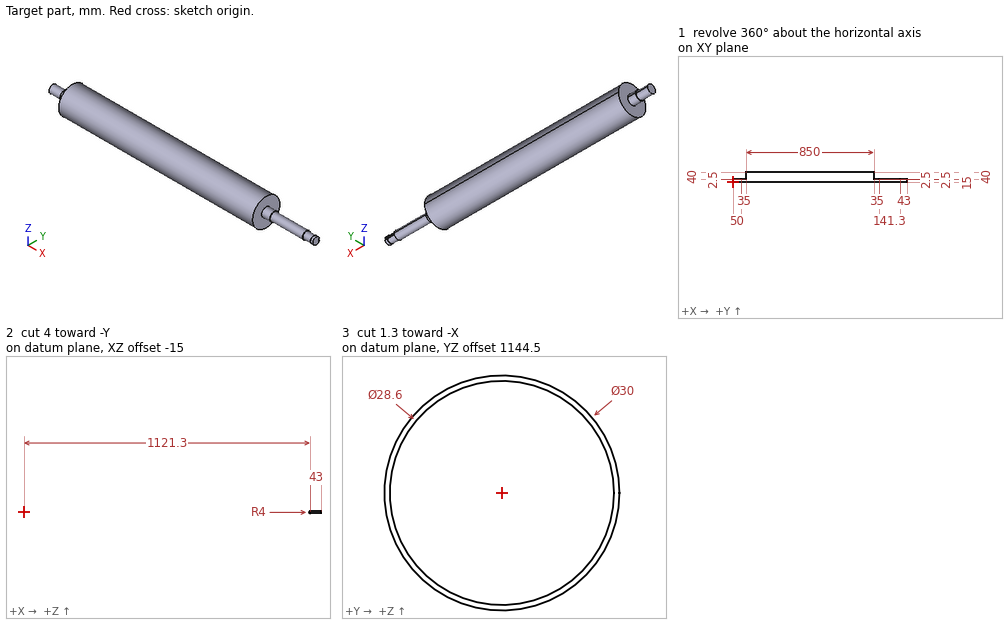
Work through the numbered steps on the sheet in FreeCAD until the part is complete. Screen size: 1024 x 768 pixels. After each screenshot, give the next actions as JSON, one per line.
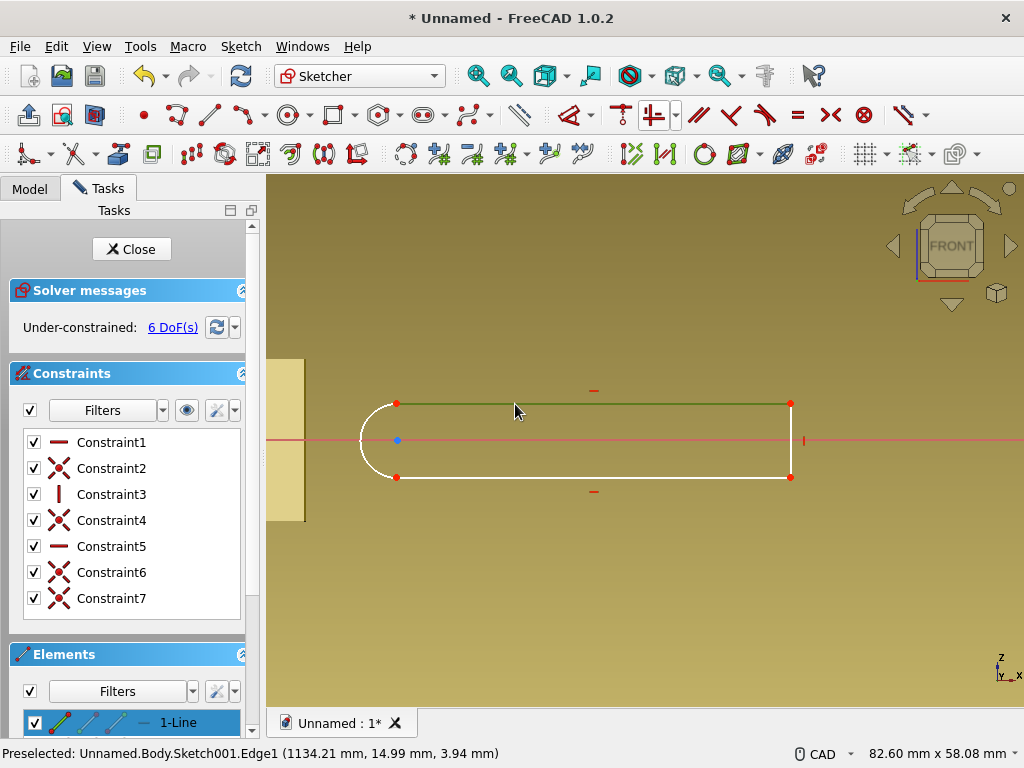
{"action": "left_click", "coordinate": [367, 419]}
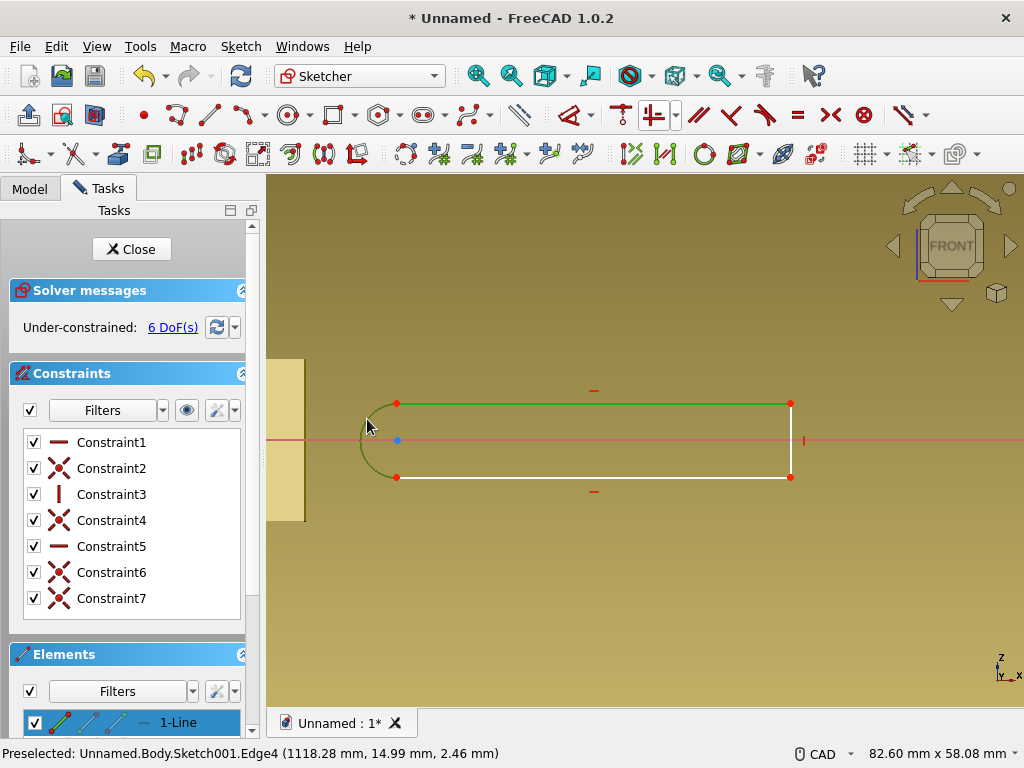
{"action": "left_click", "coordinate": [765, 116]}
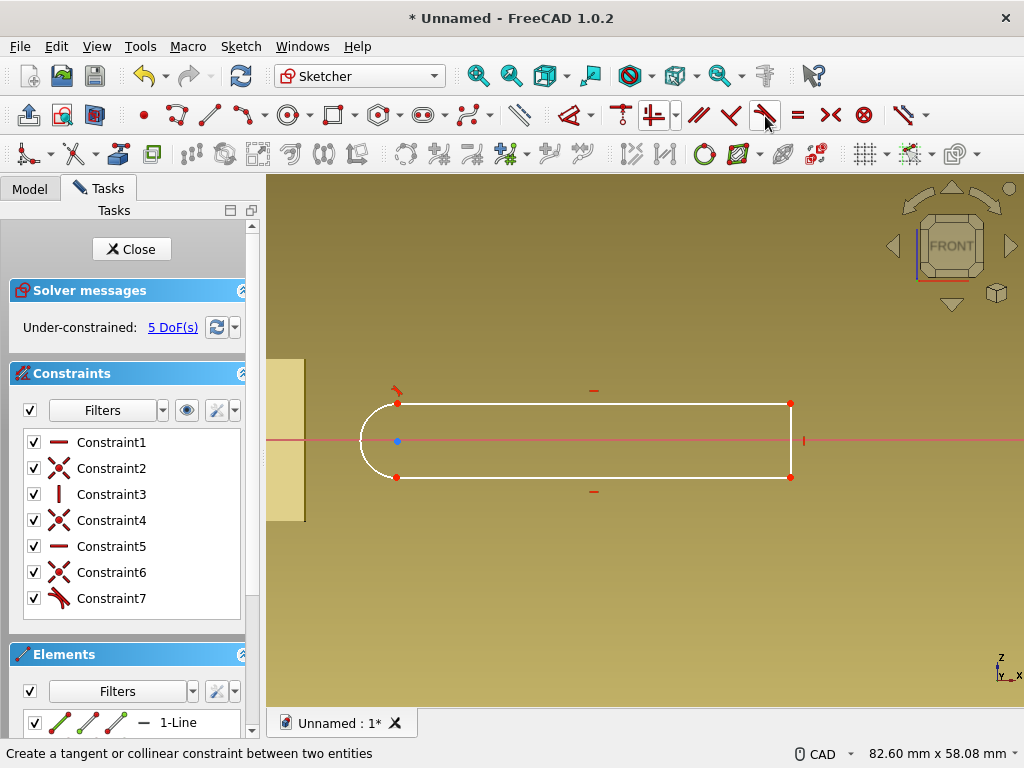
{"action": "left_click", "coordinate": [673, 478]}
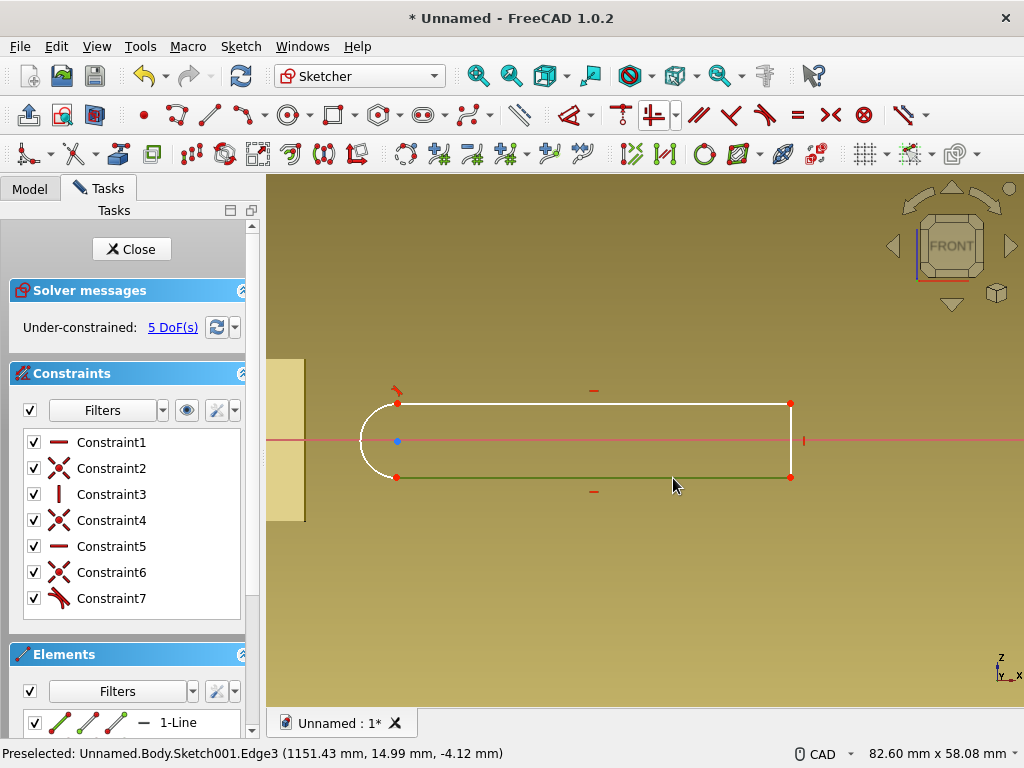
{"action": "left_click", "coordinate": [368, 419]}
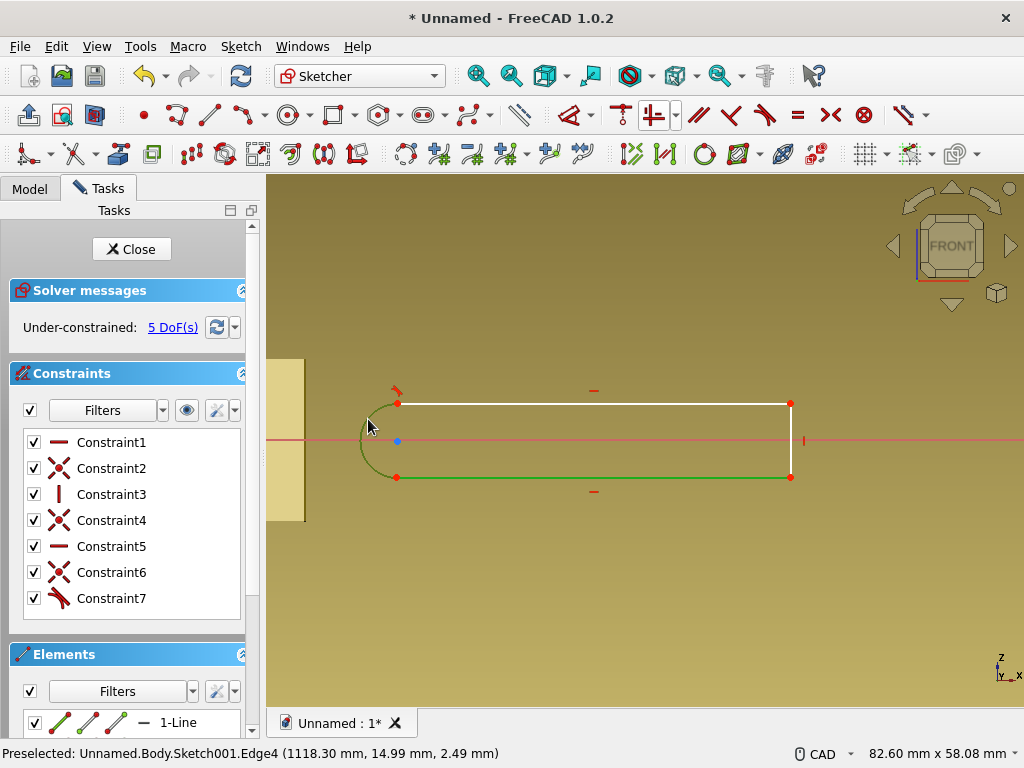
{"action": "key", "text": "t"}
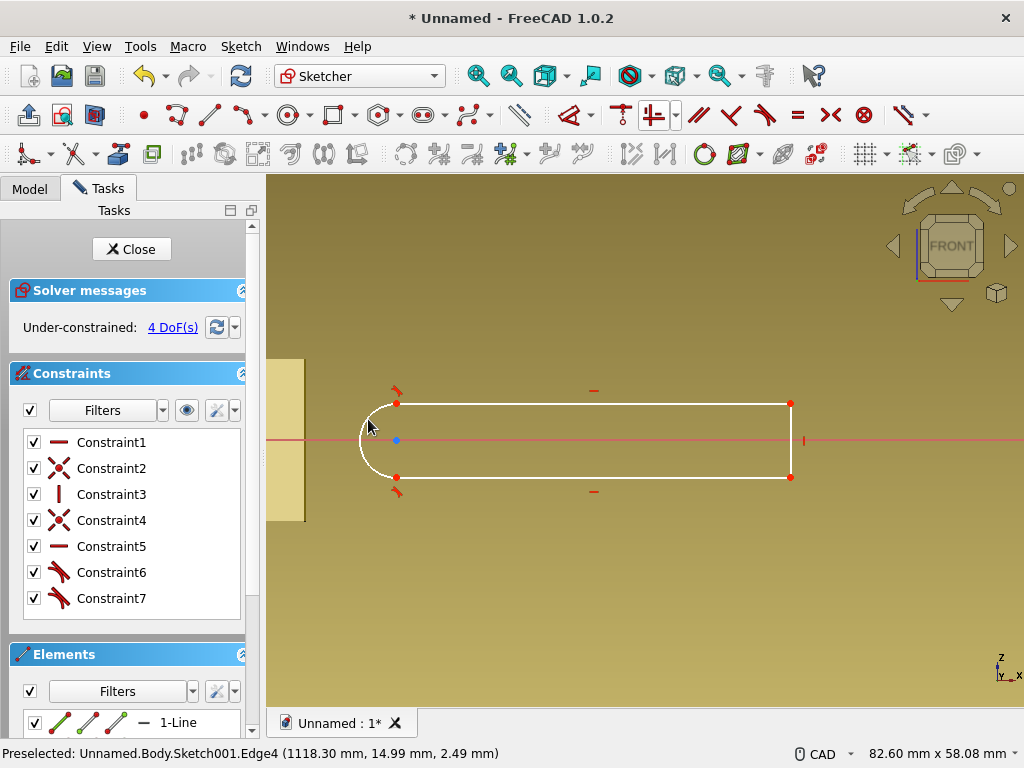
{"action": "left_click", "coordinate": [397, 441]}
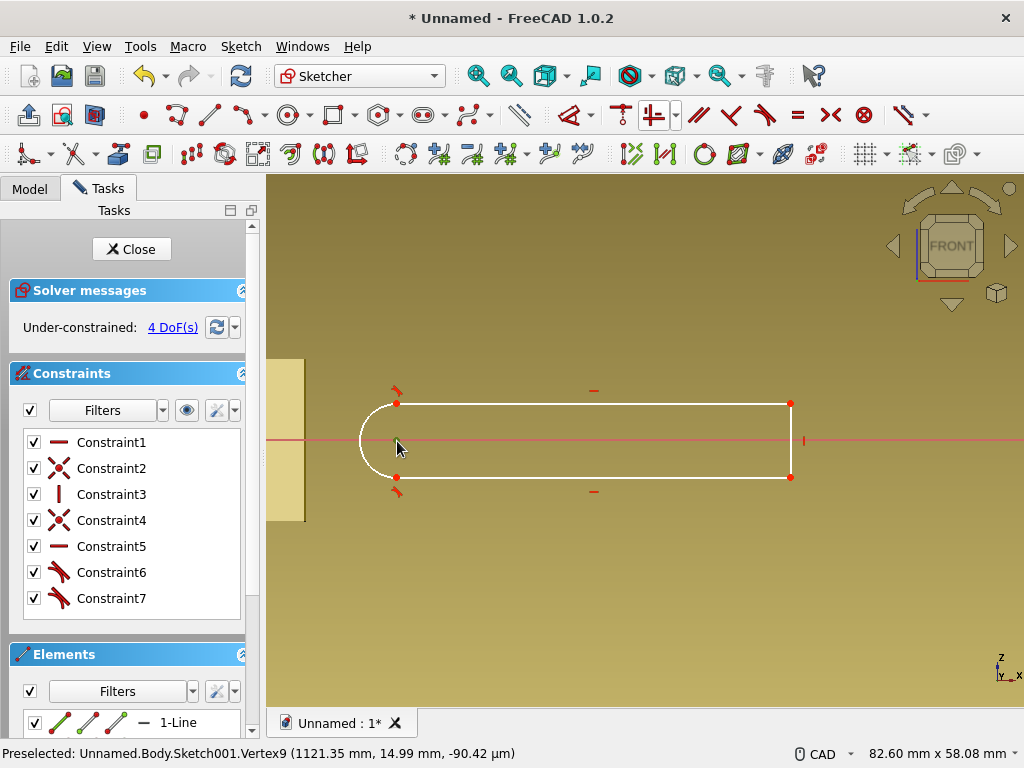
{"action": "left_click", "coordinate": [415, 440]}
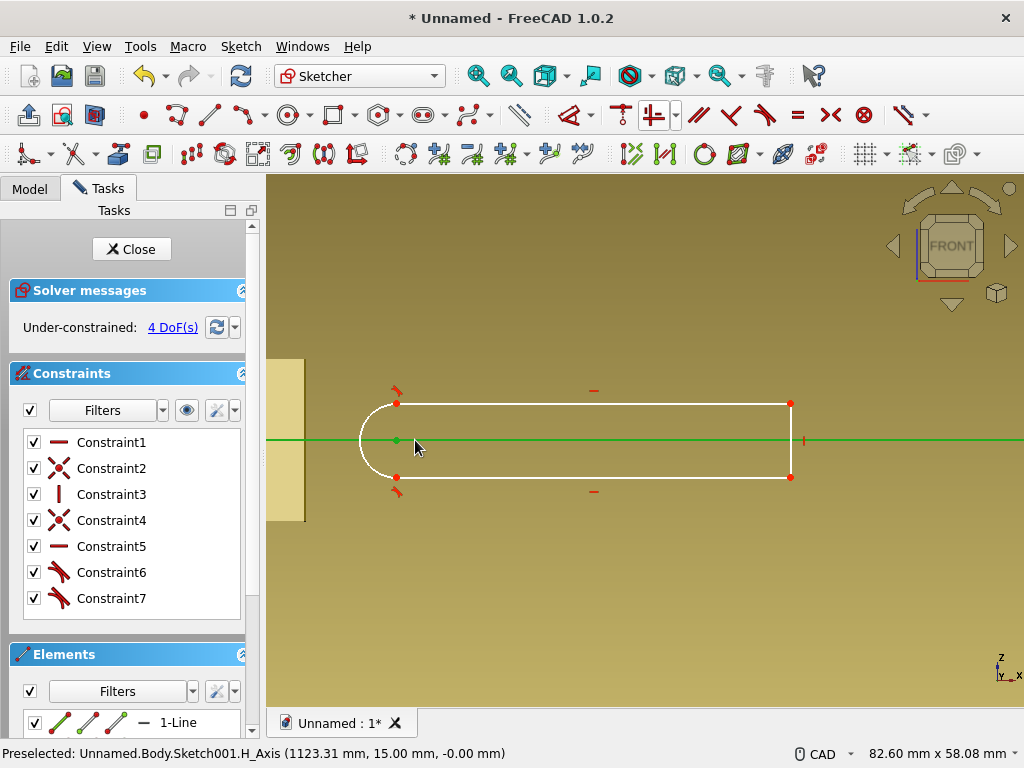
{"action": "key", "text": "c"}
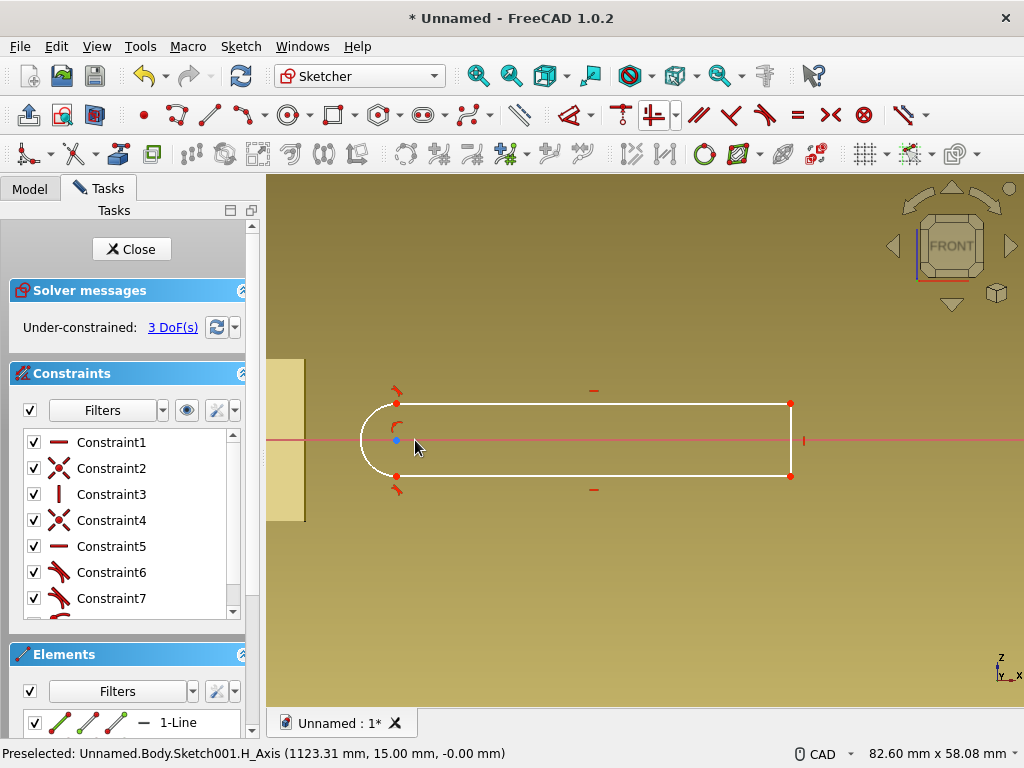
{"action": "key", "text": "d"}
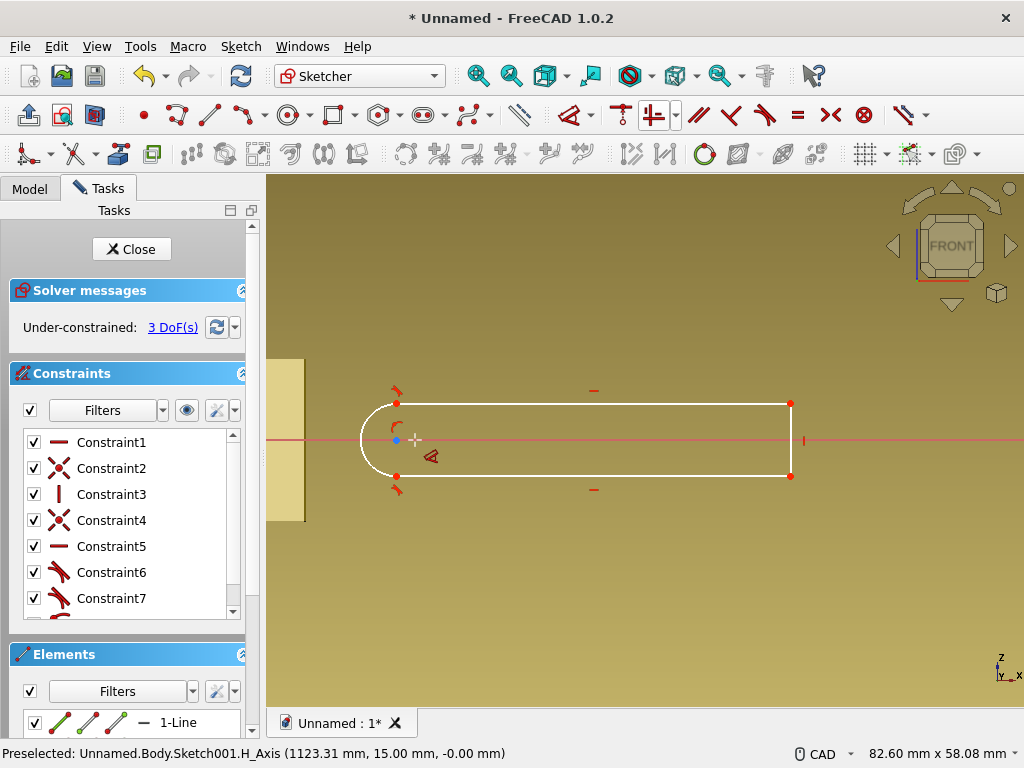
{"action": "left_click", "coordinate": [368, 419]}
{"action": "left_click", "coordinate": [342, 400]}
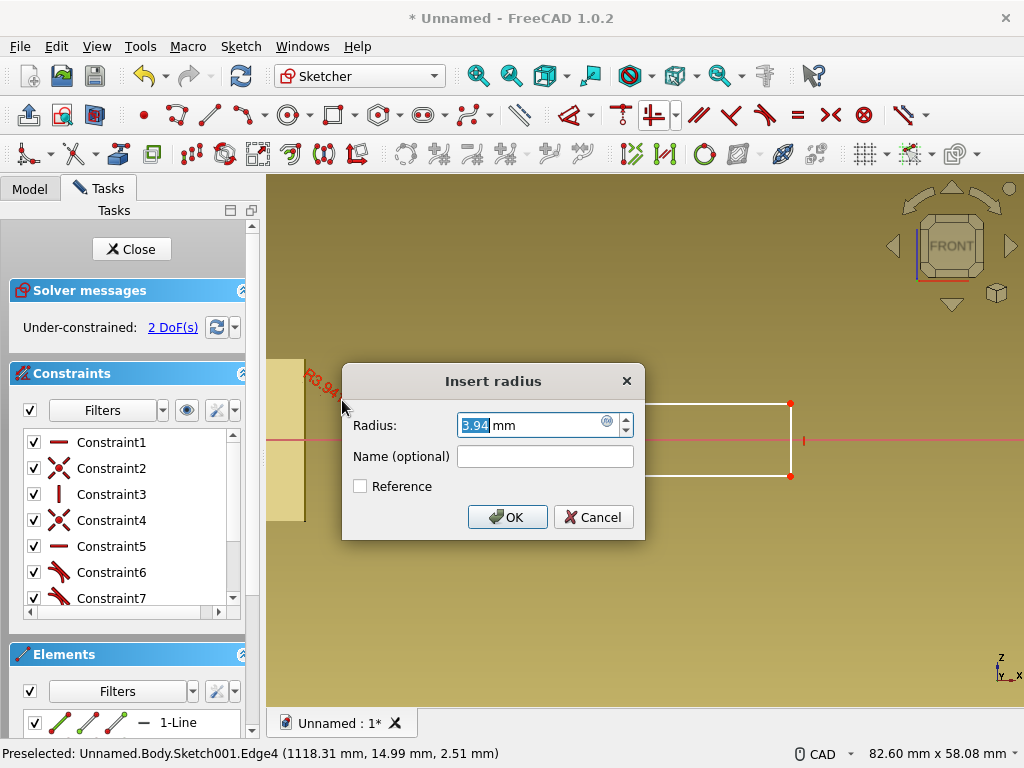
{"action": "type", "text": "4"}
{"action": "key", "text": "Return"}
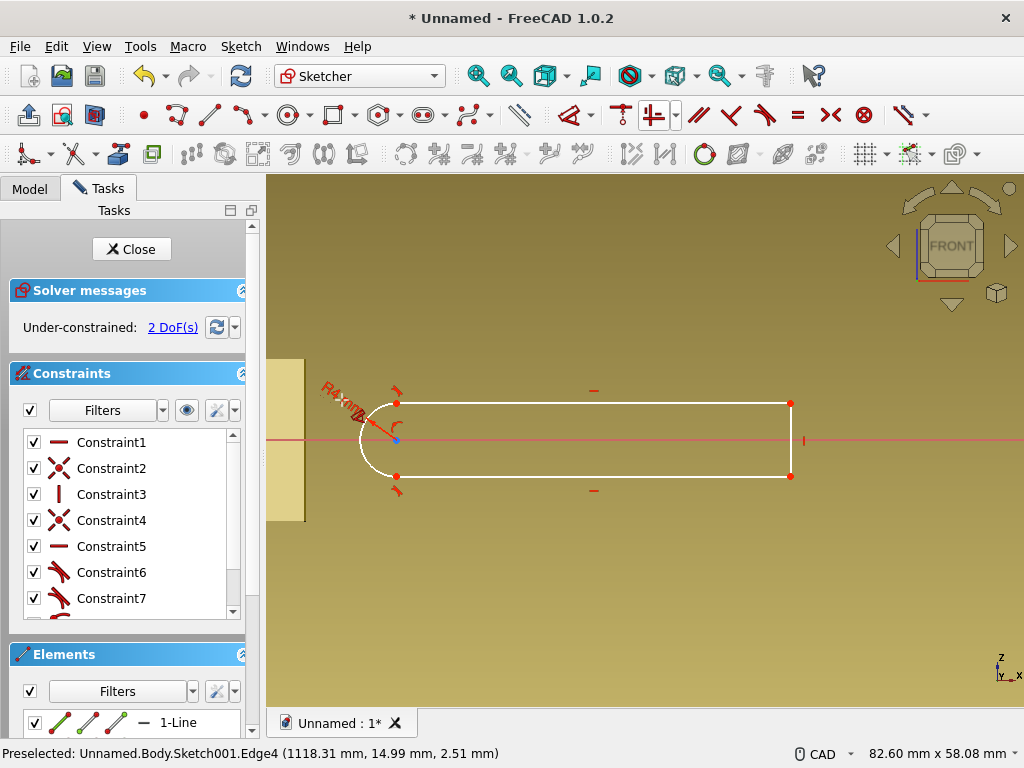
{"action": "left_click", "coordinate": [515, 403]}
{"action": "left_click", "coordinate": [594, 369]}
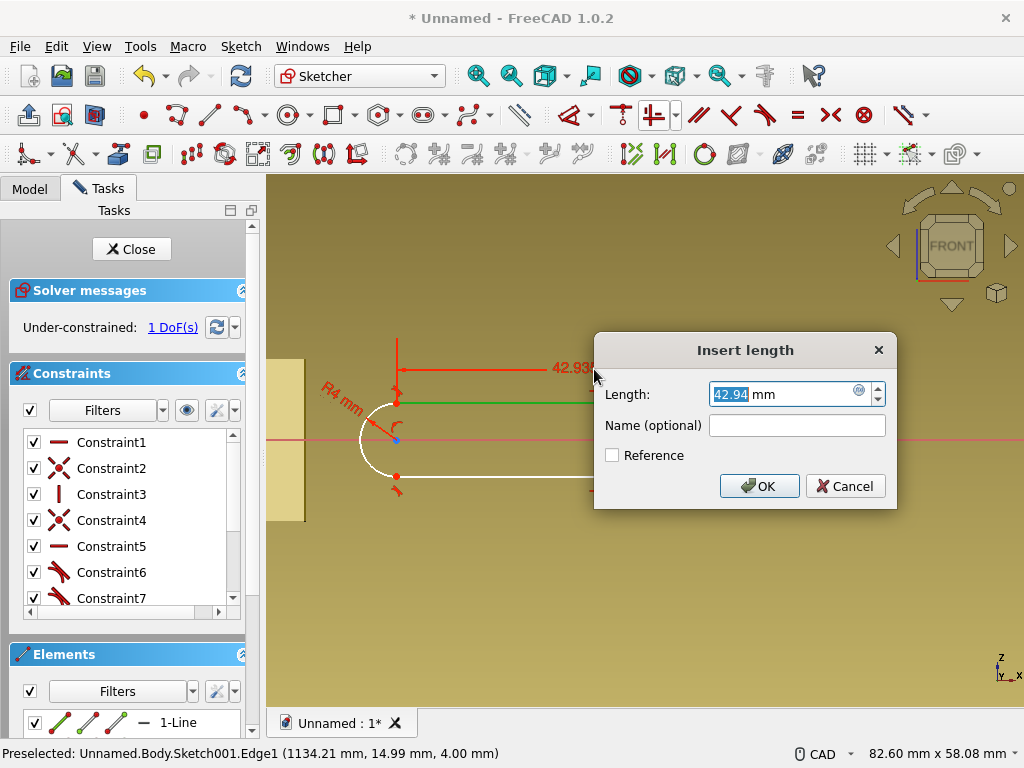
{"action": "type", "text": "43"}
{"action": "key", "text": "Return"}